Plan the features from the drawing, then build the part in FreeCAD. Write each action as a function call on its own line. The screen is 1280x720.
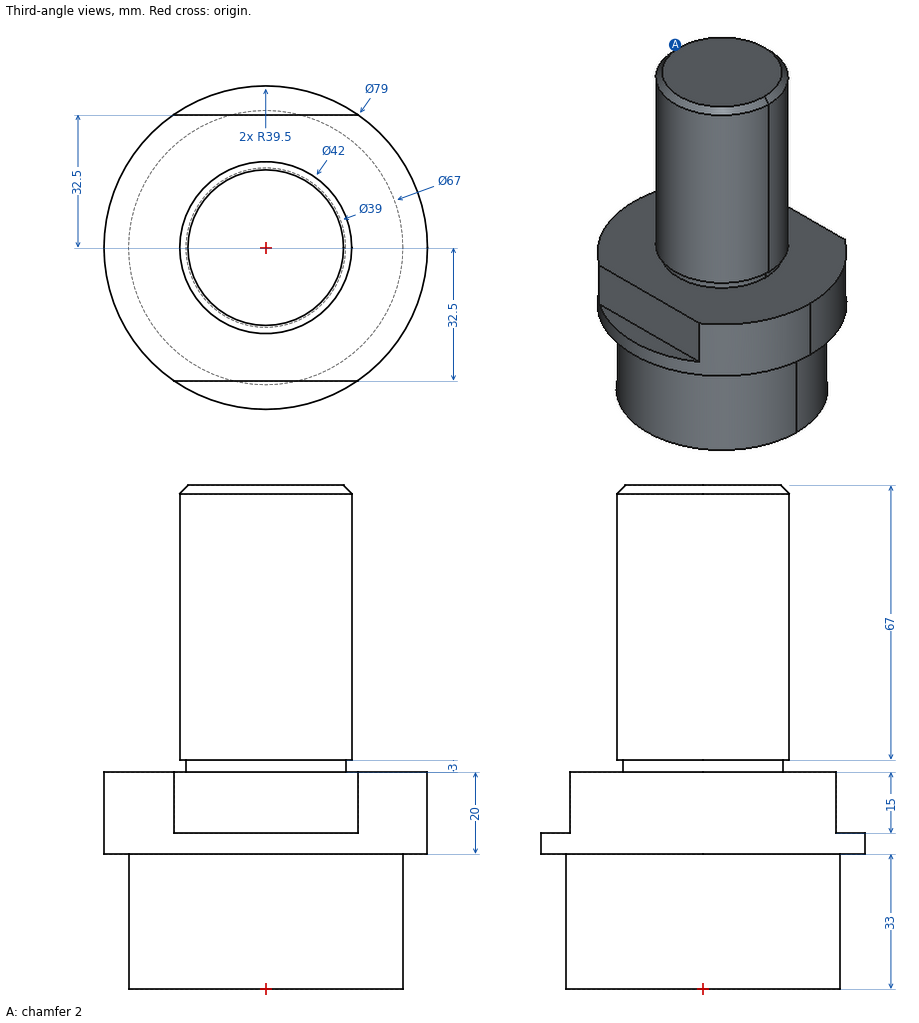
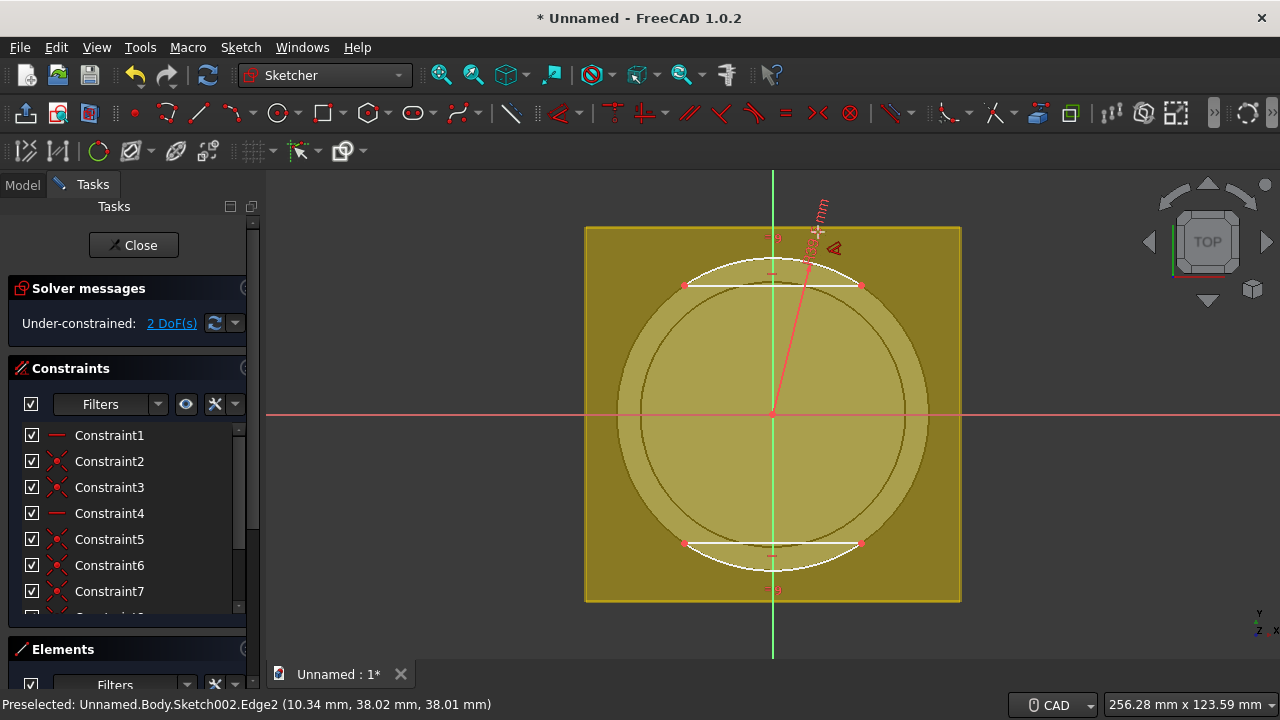
click(684, 286)
click(650, 350)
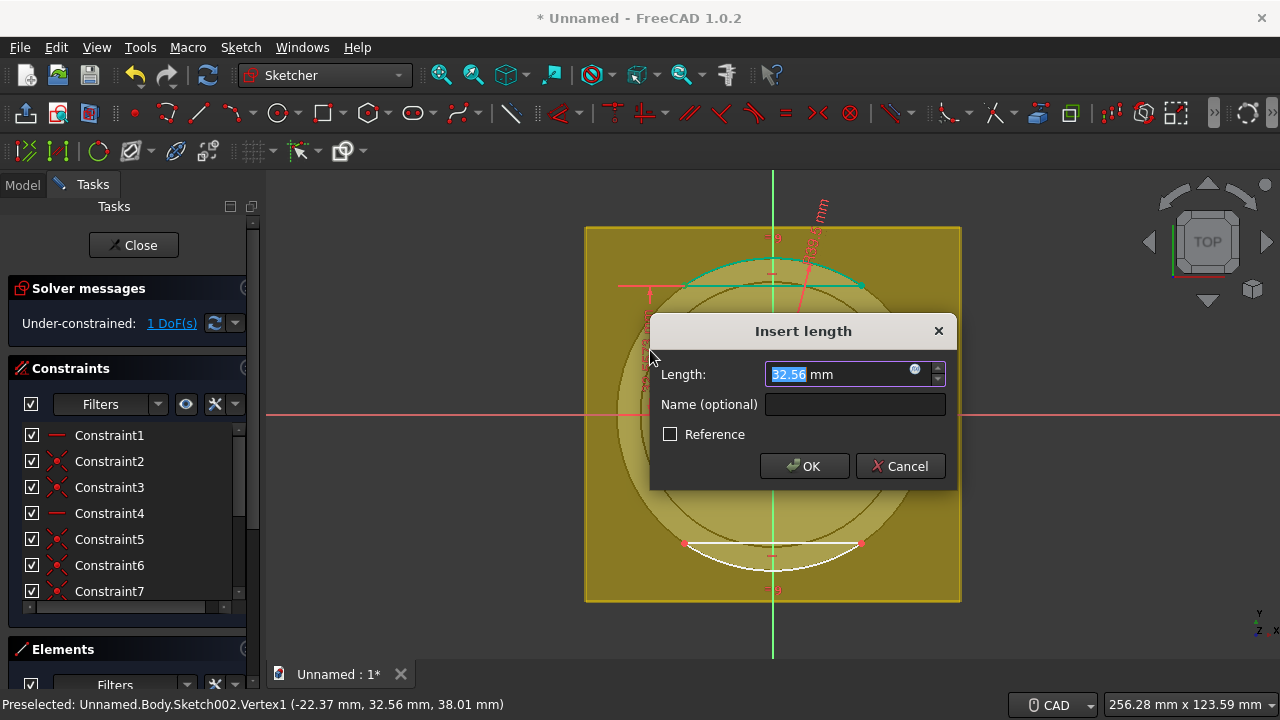
text(32.5)
key(Return)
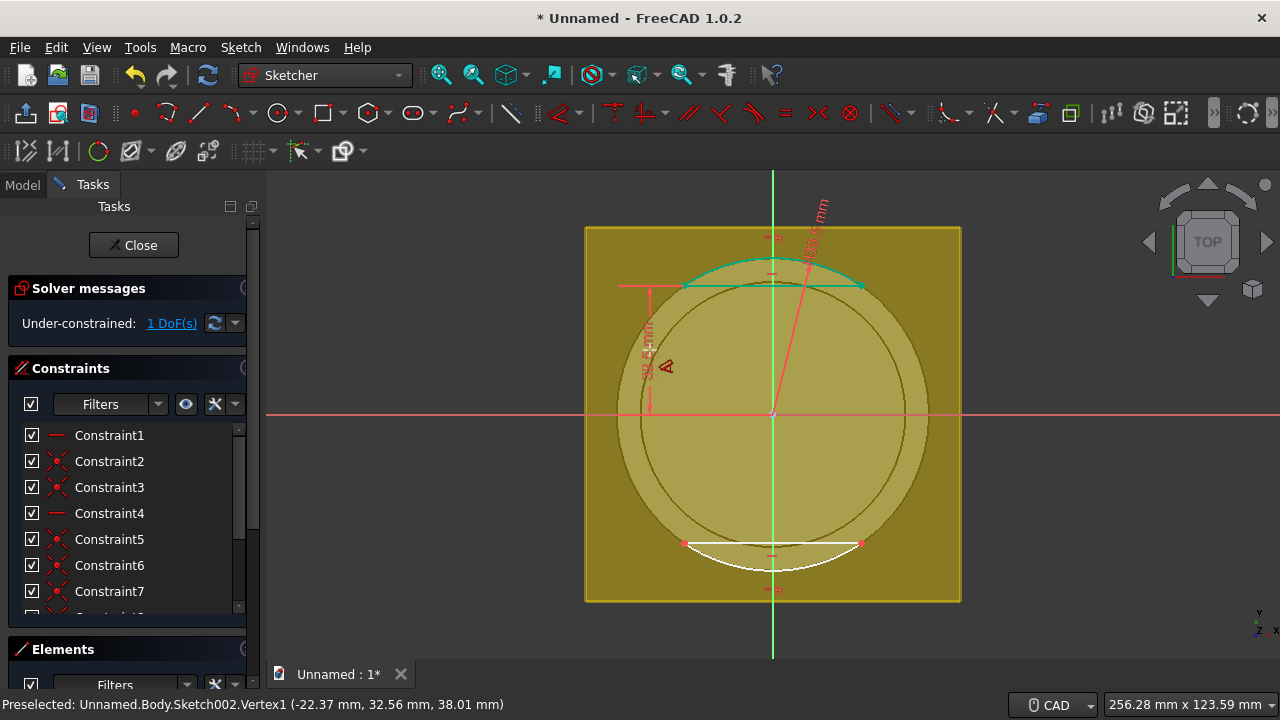
click(862, 543)
click(896, 479)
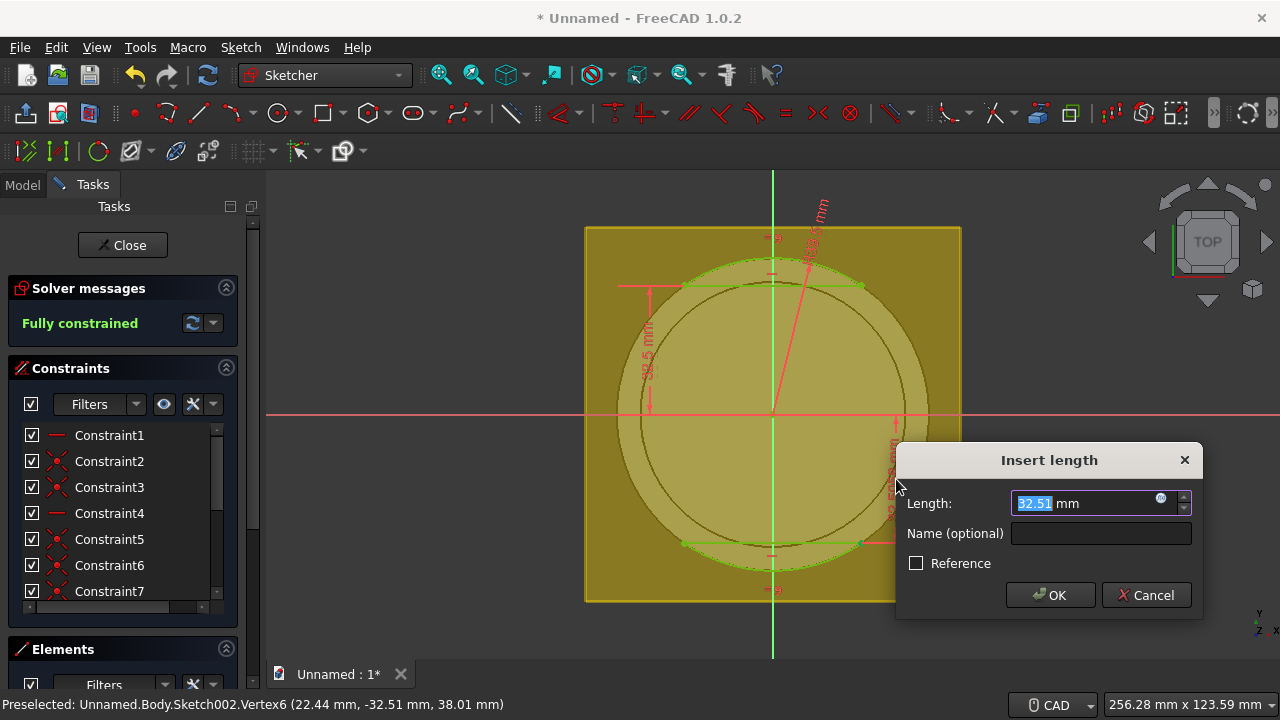
text(32.5)
key(Return)
key(Escape)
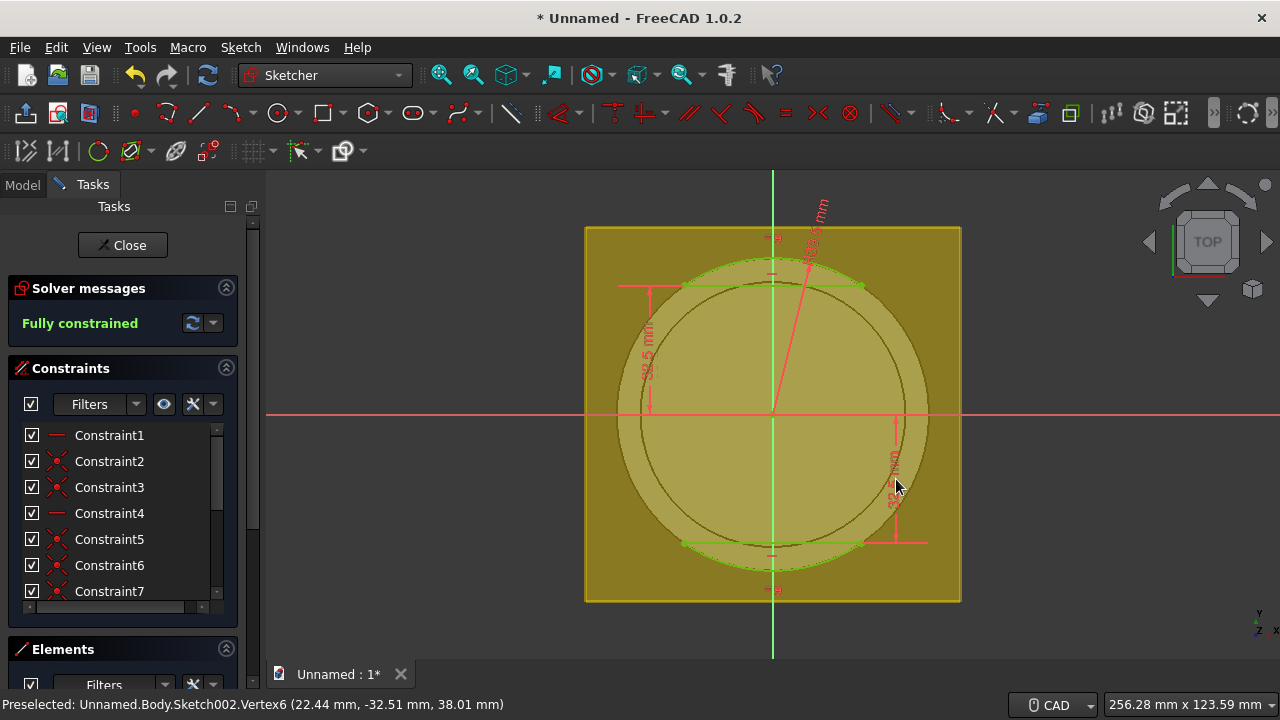
click(123, 245)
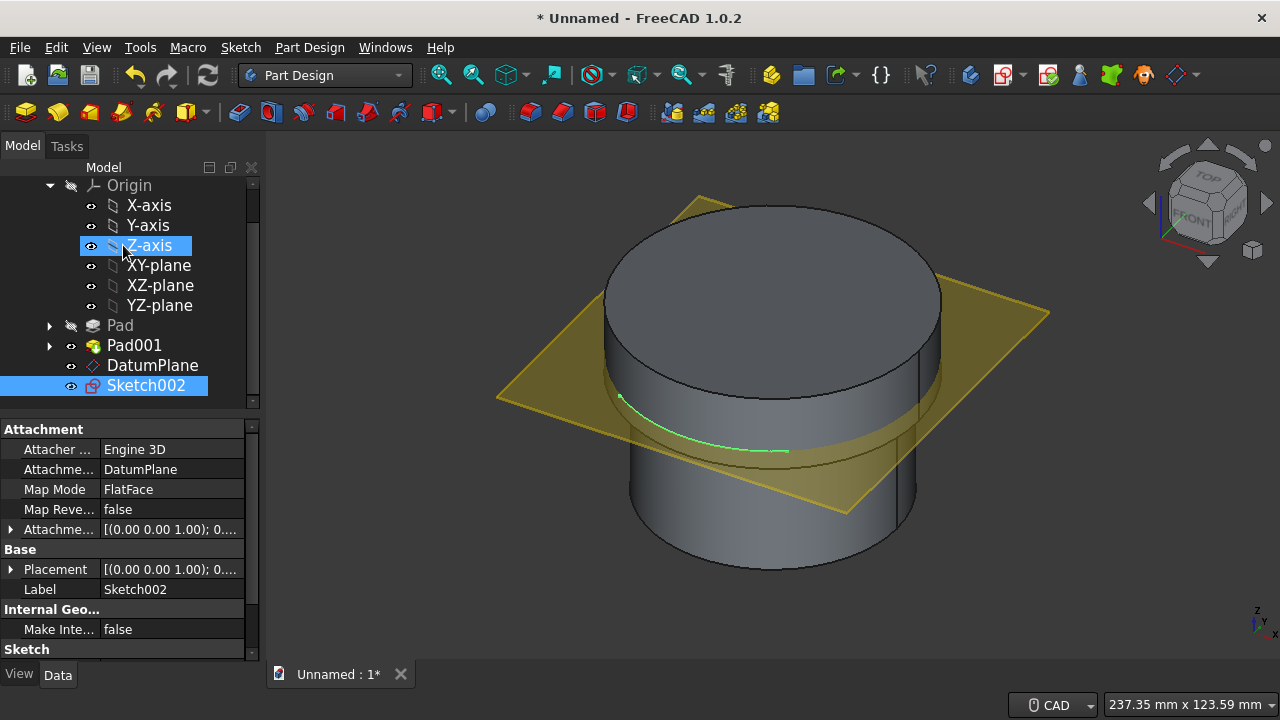
click(240, 112)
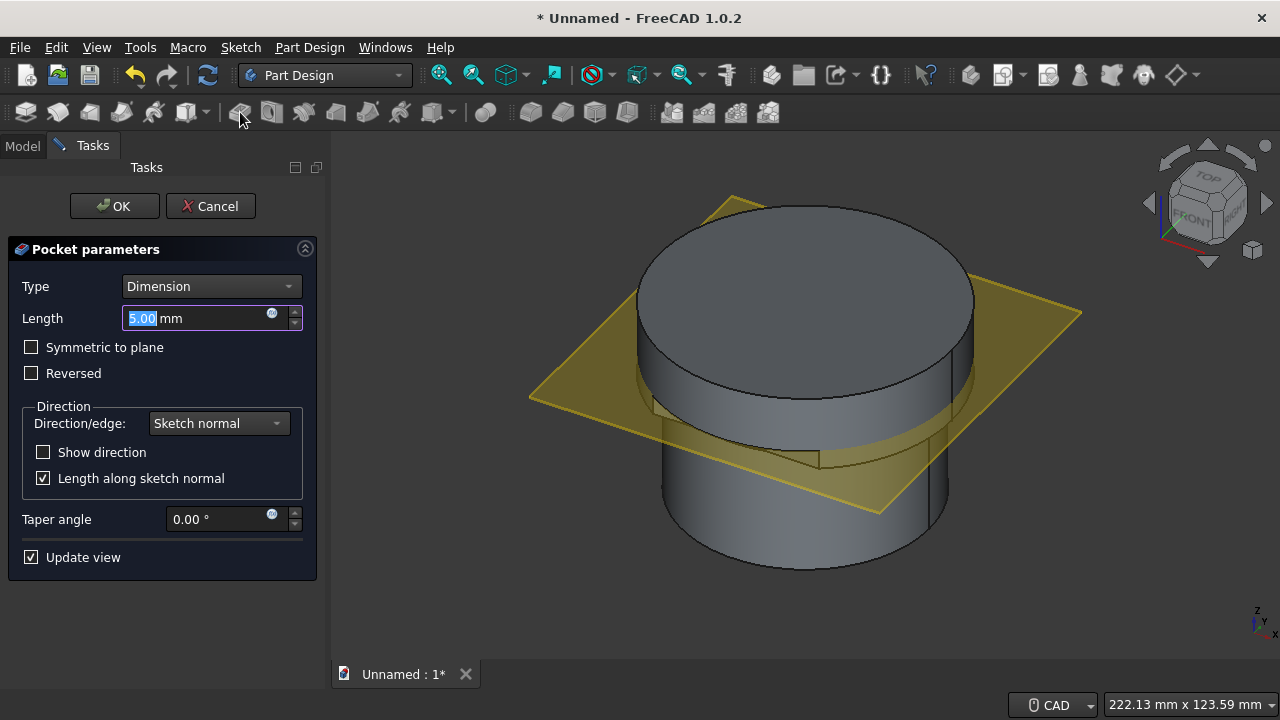
text(15)
key(Tab)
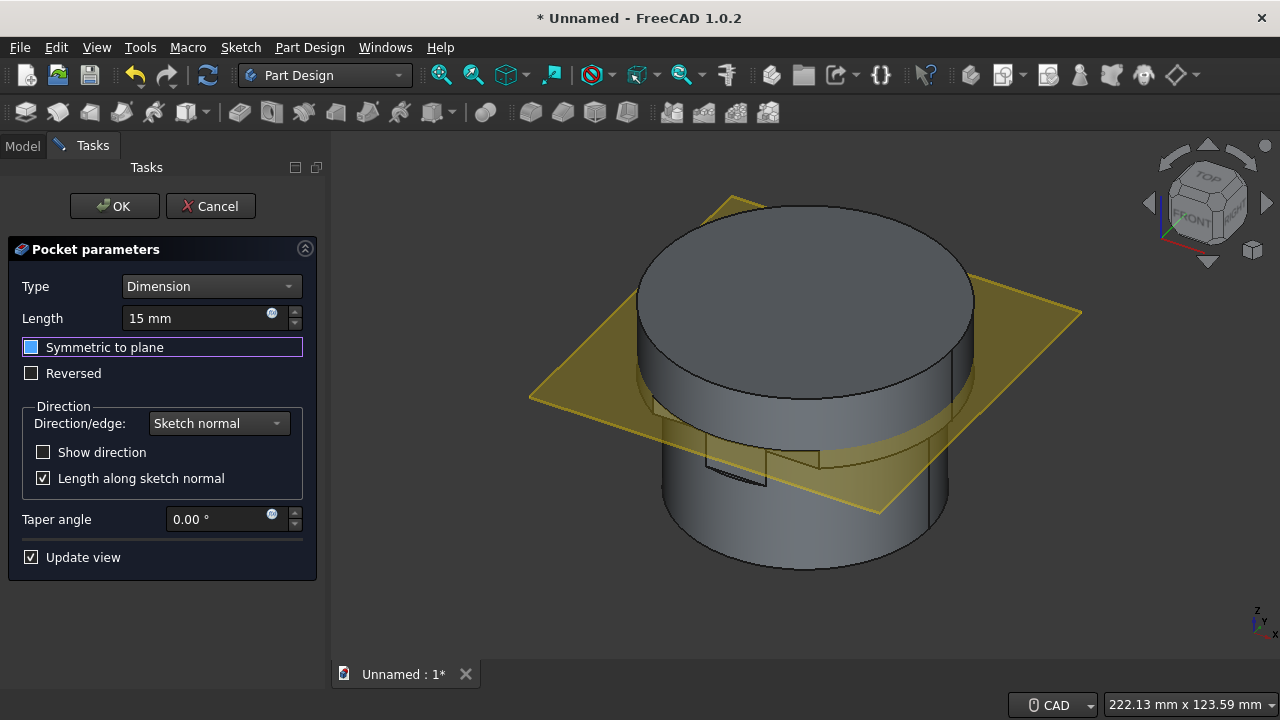
click(30, 373)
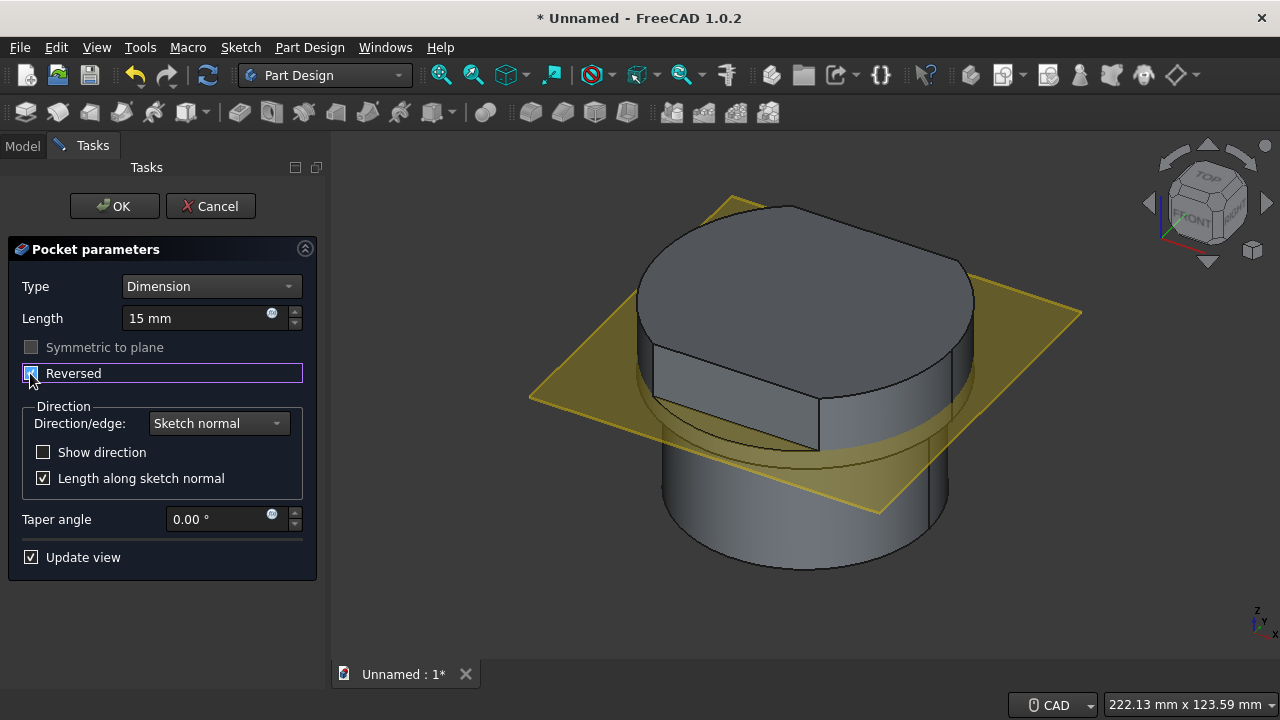
click(115, 206)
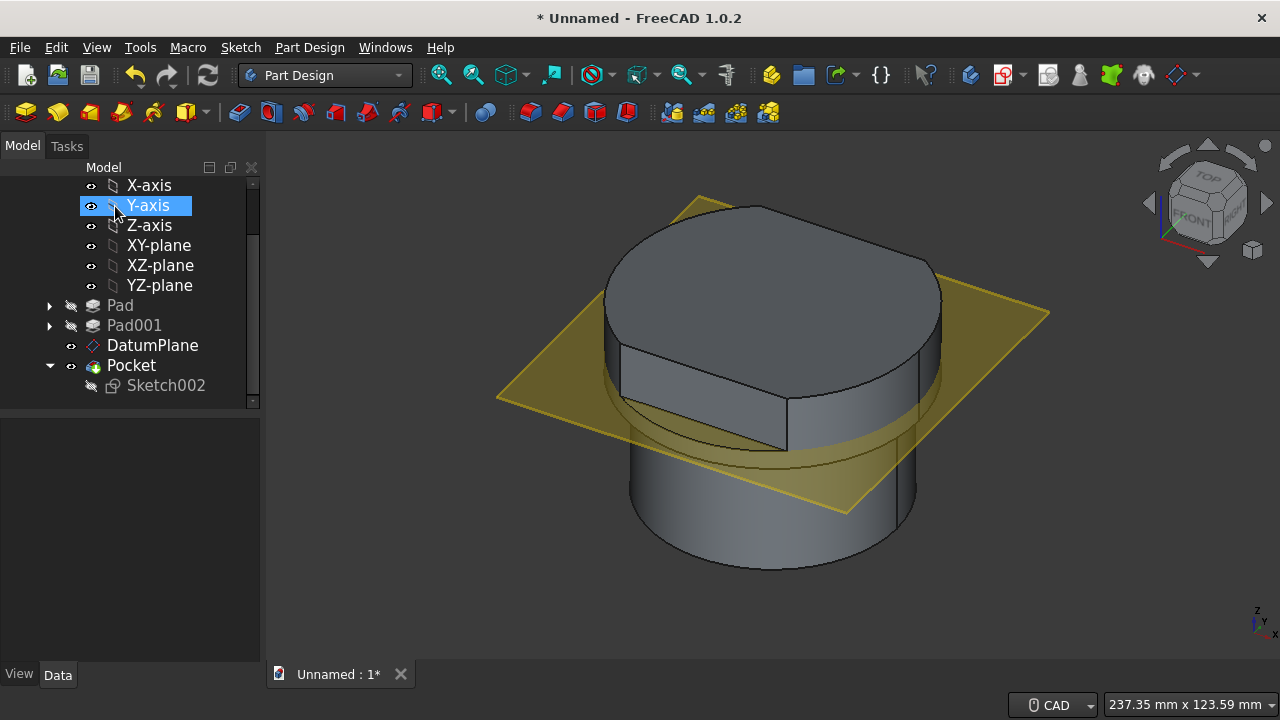
click(116, 346)
key(space)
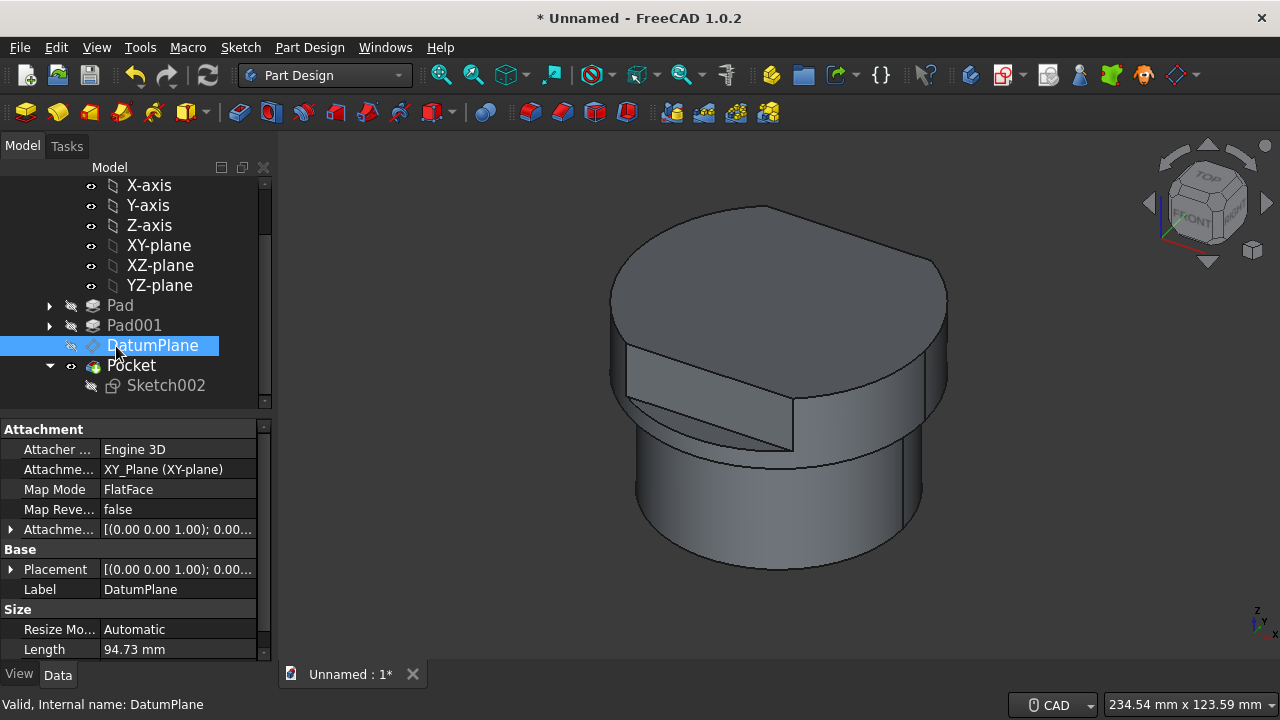
click(779, 301)